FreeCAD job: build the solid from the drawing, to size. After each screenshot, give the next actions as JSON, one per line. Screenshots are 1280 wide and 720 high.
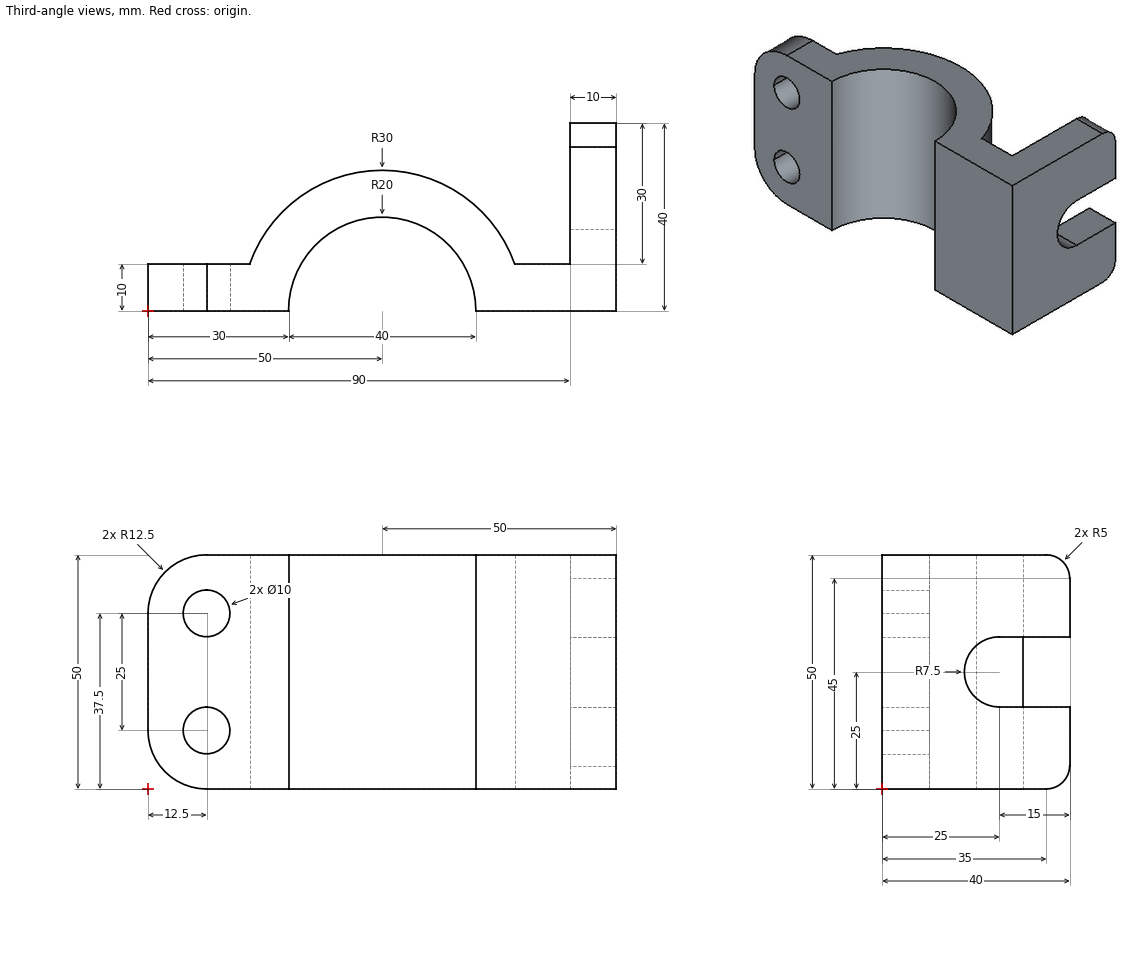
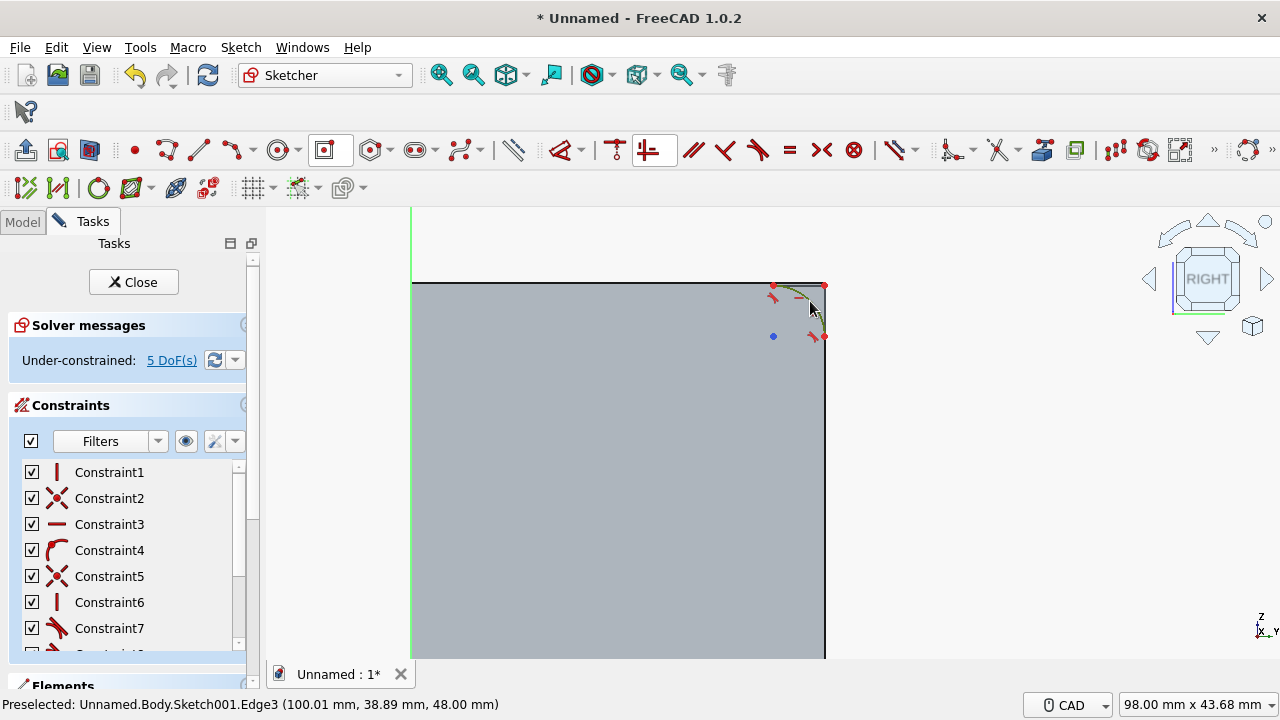
{"action": "scroll", "coordinate": [810, 300], "scroll_direction": "down", "scroll_amount": 3}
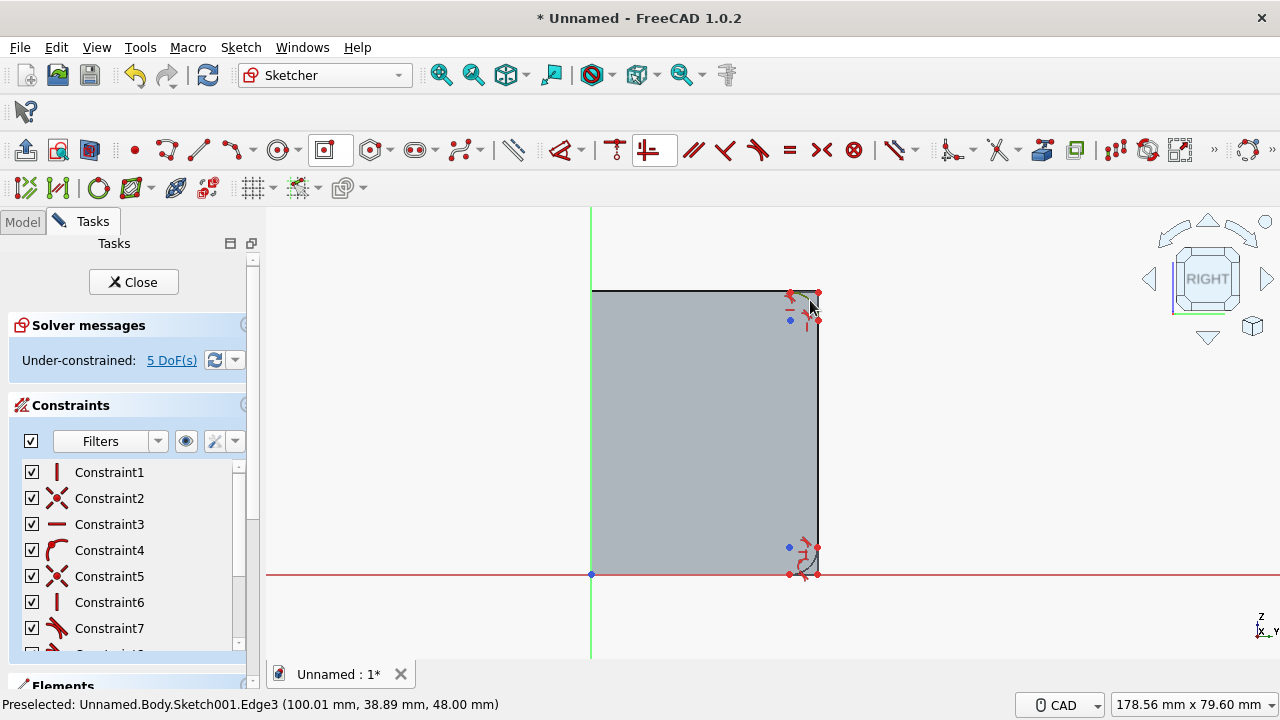
{"action": "scroll", "coordinate": [810, 567], "scroll_direction": "up", "scroll_amount": 3}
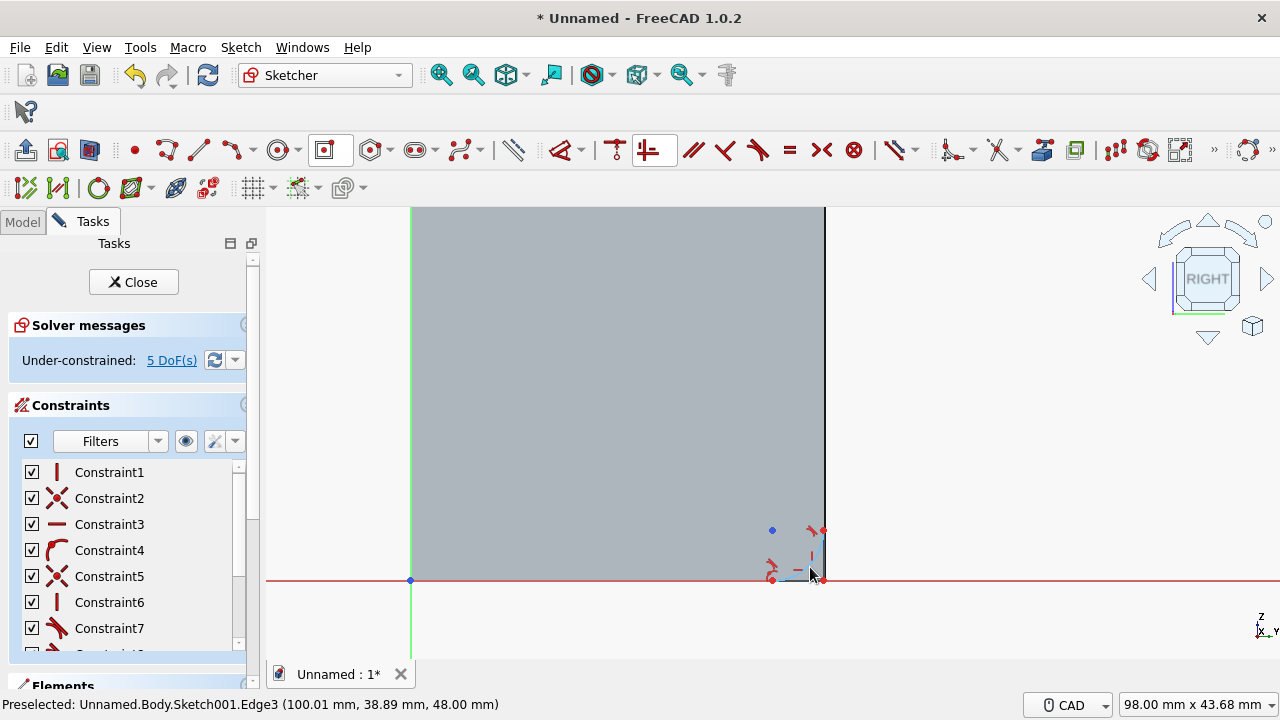
{"action": "left_click", "coordinate": [809, 566]}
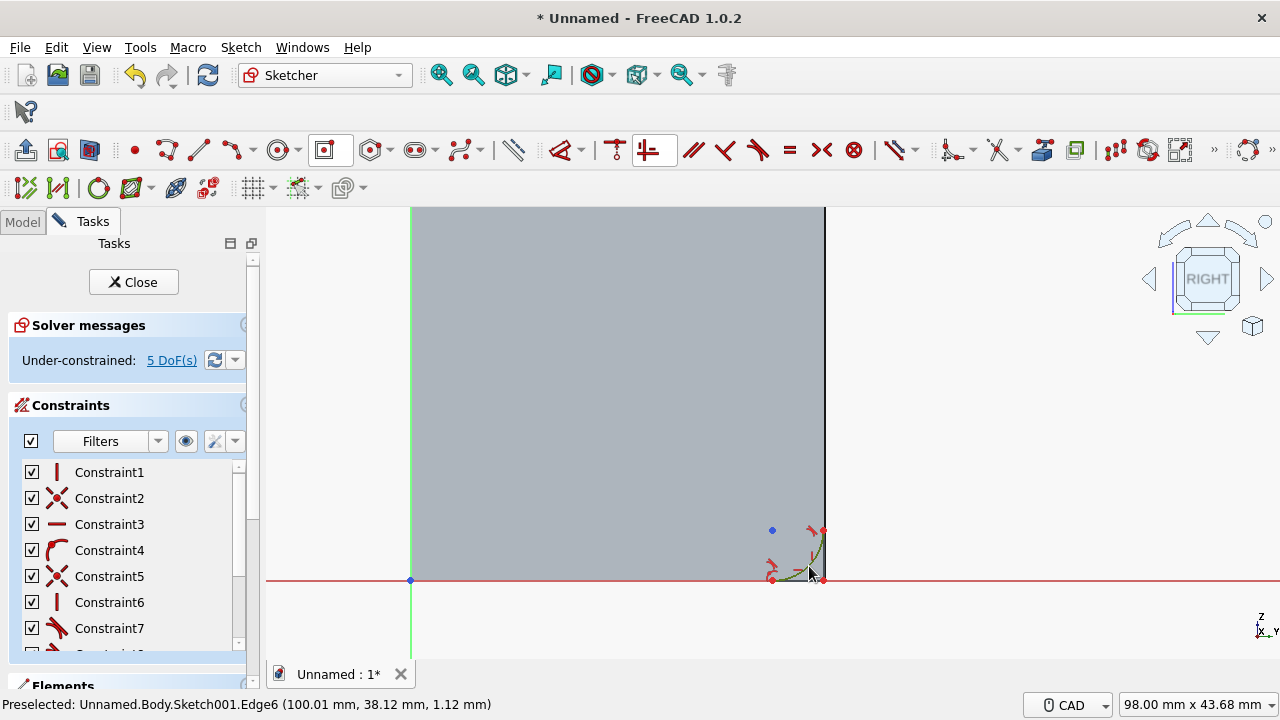
{"action": "left_click", "coordinate": [790, 150]}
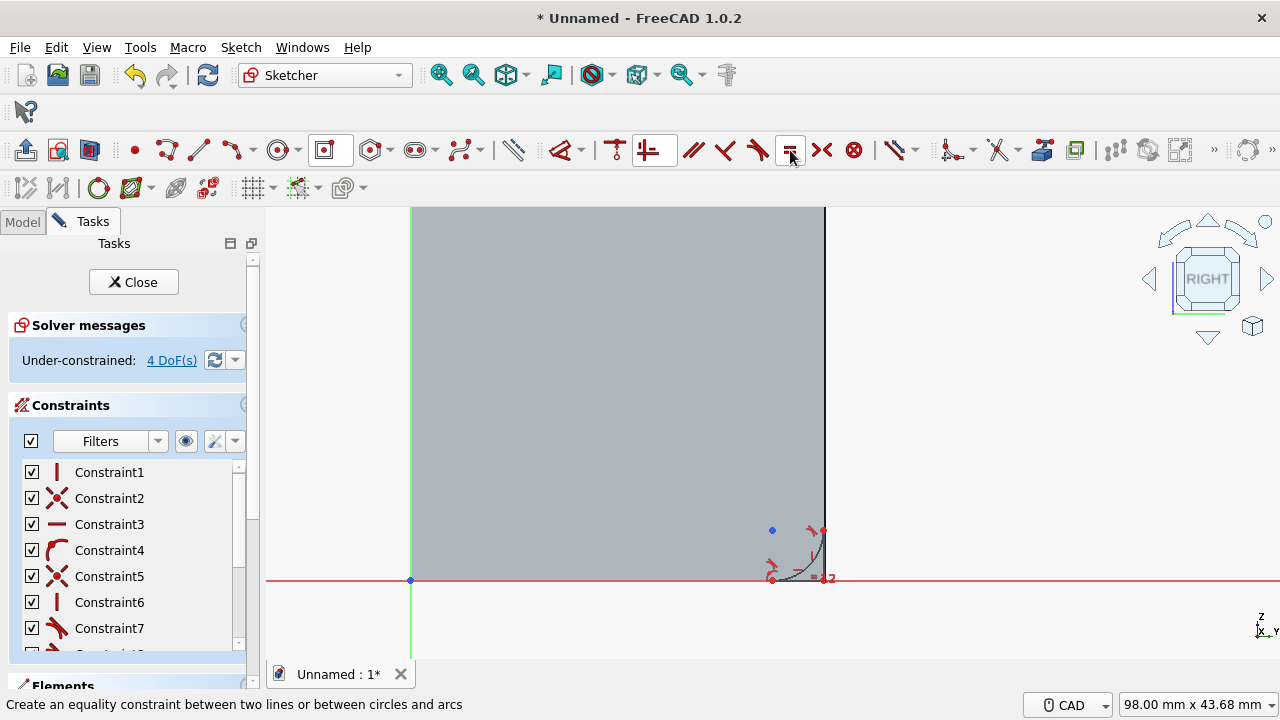
{"action": "left_click", "coordinate": [560, 150]}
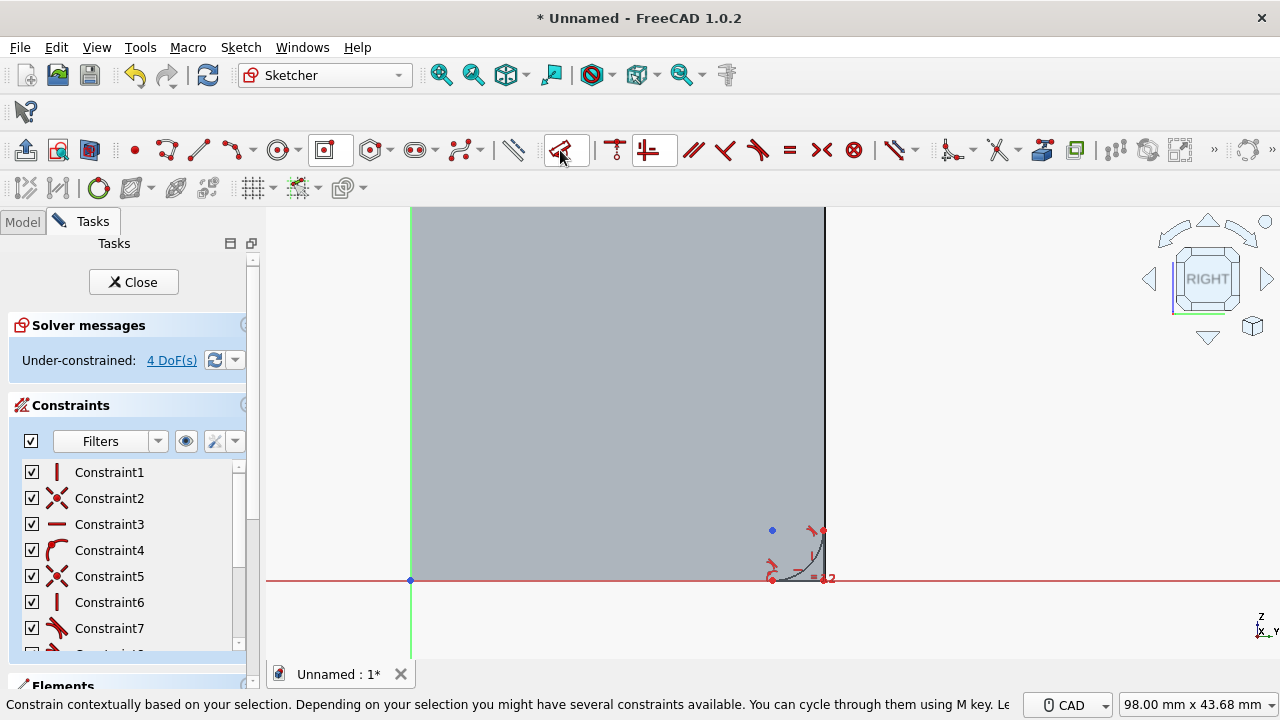
{"action": "scroll", "coordinate": [810, 568], "scroll_direction": "down", "scroll_amount": 3}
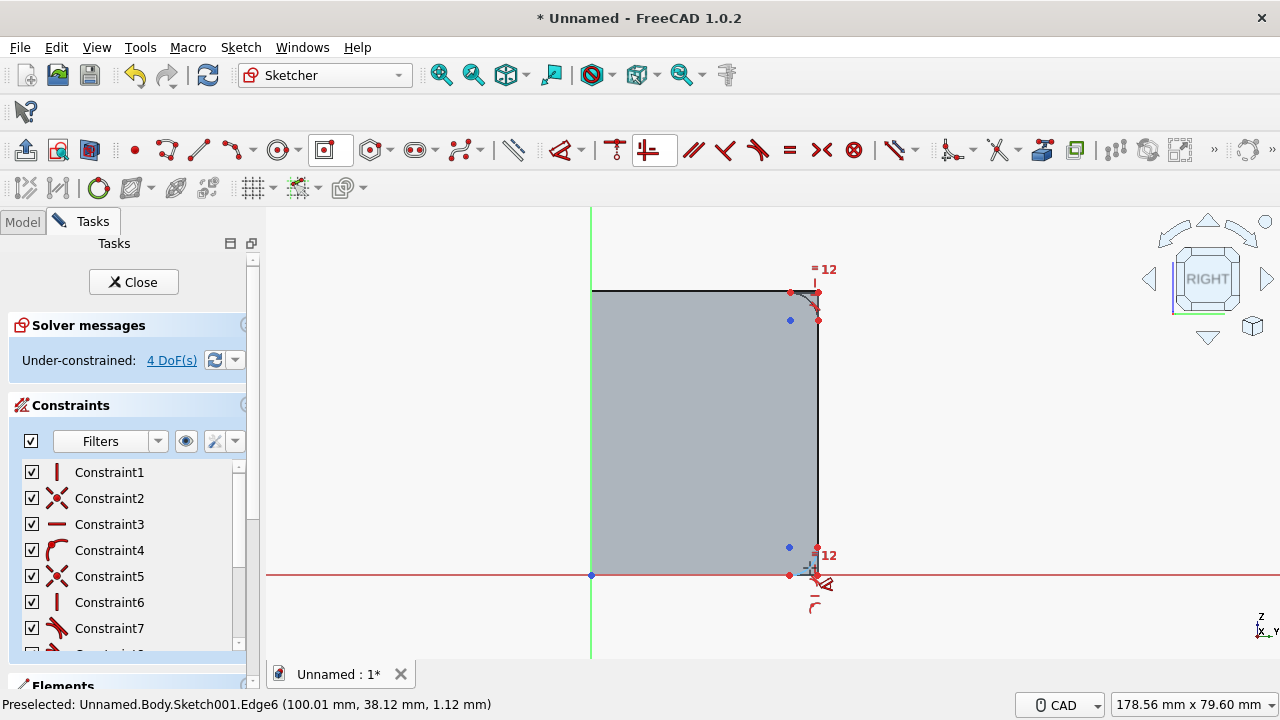
{"action": "scroll", "coordinate": [810, 301], "scroll_direction": "up", "scroll_amount": 3}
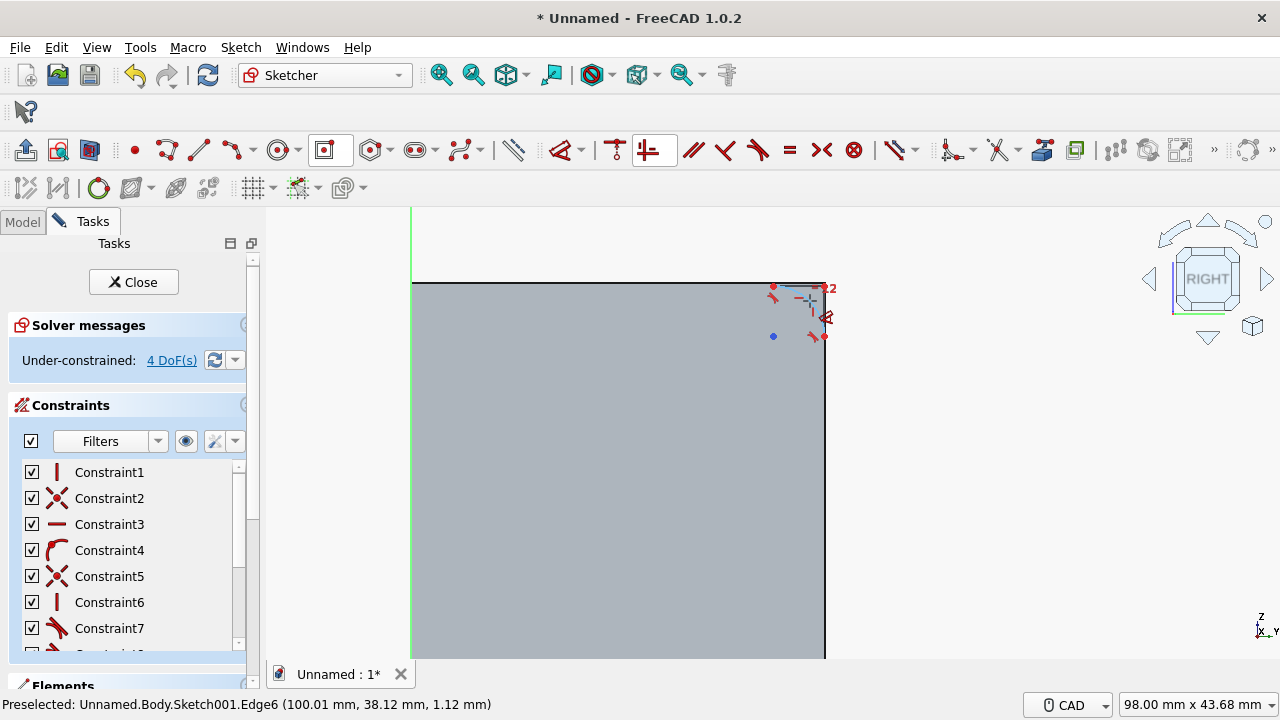
{"action": "left_click", "coordinate": [810, 301]}
{"action": "left_click", "coordinate": [853, 314]}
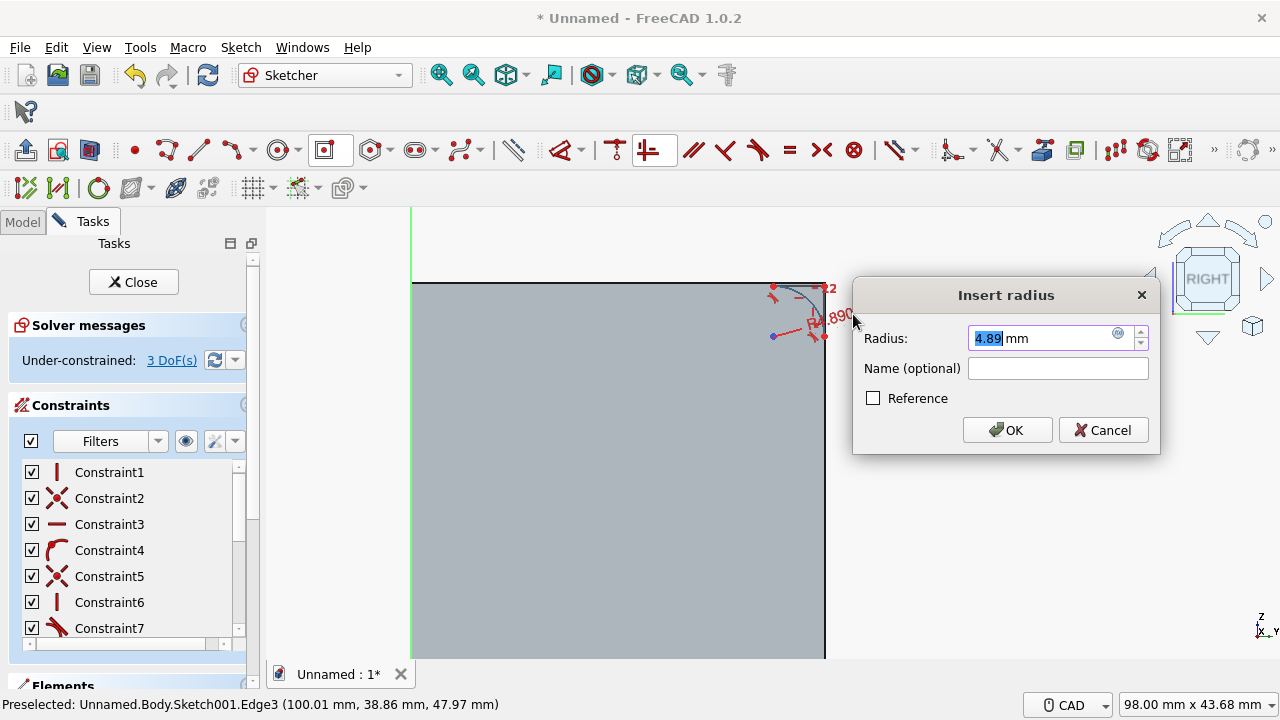
{"action": "type", "text": "5"}
{"action": "key", "text": "Return"}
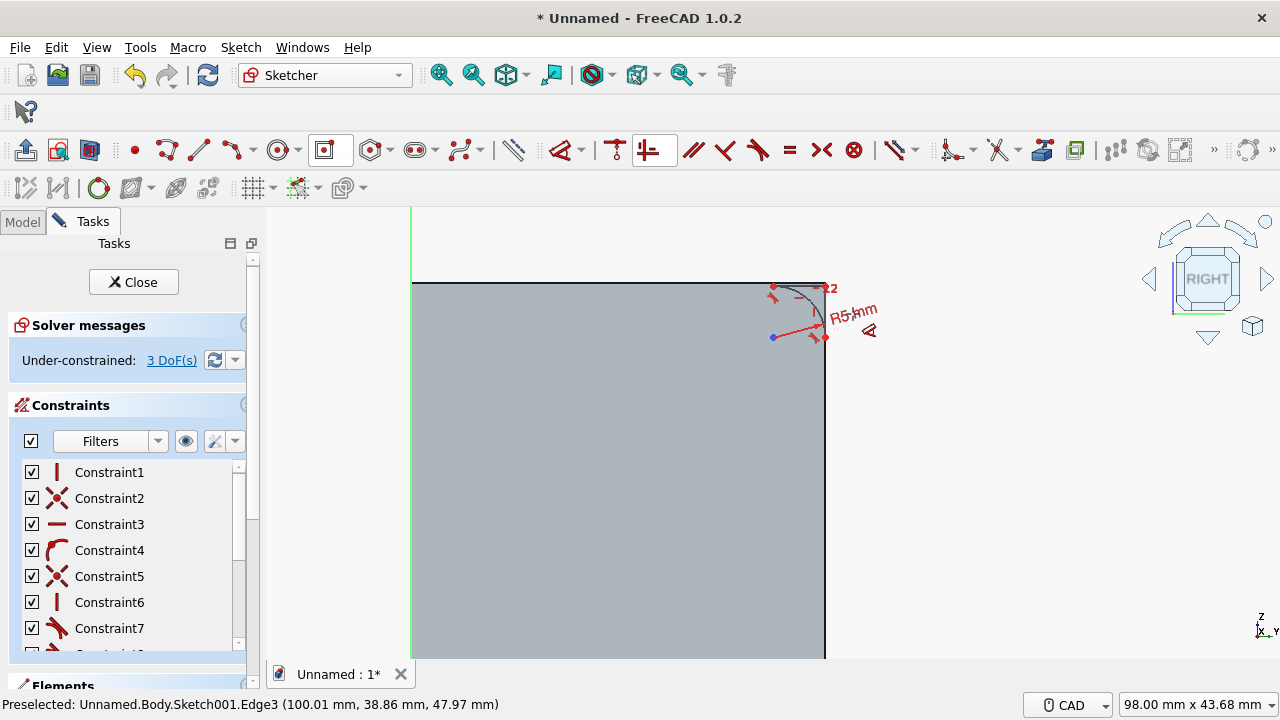
{"action": "left_click", "coordinate": [825, 338]}
{"action": "left_click", "coordinate": [618, 304]}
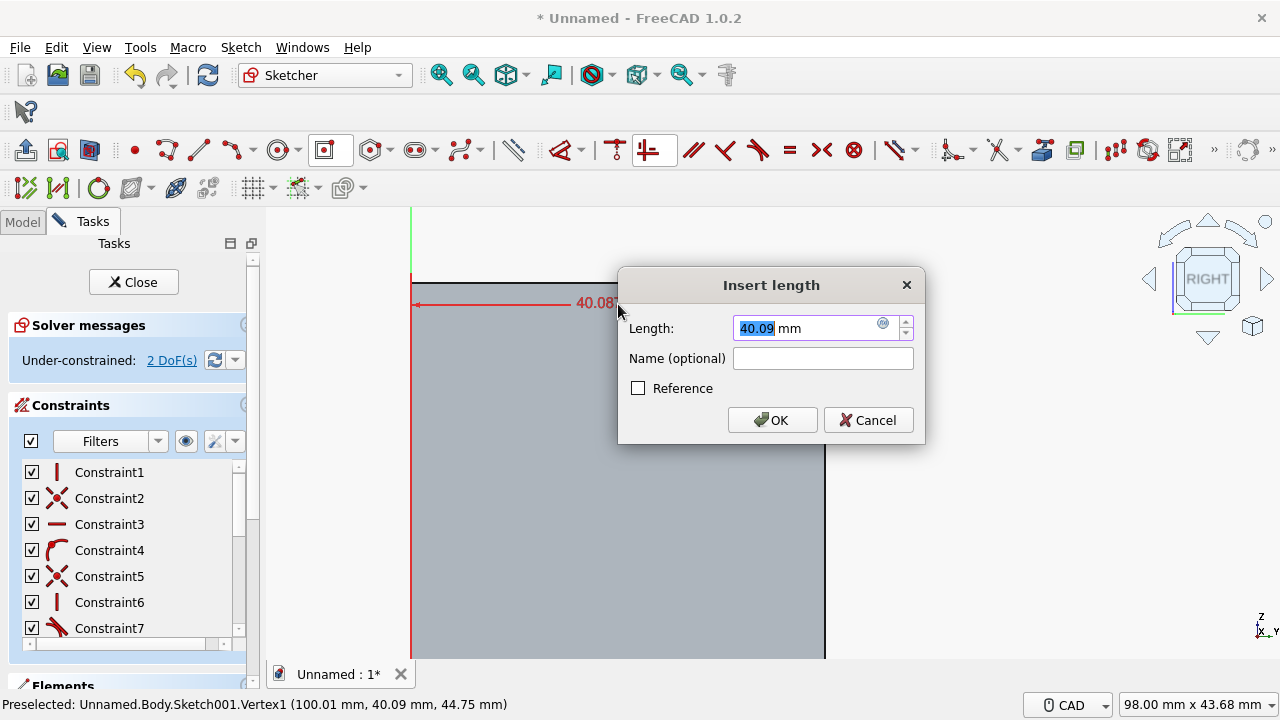
{"action": "type", "text": "40"}
{"action": "key", "text": "Return"}